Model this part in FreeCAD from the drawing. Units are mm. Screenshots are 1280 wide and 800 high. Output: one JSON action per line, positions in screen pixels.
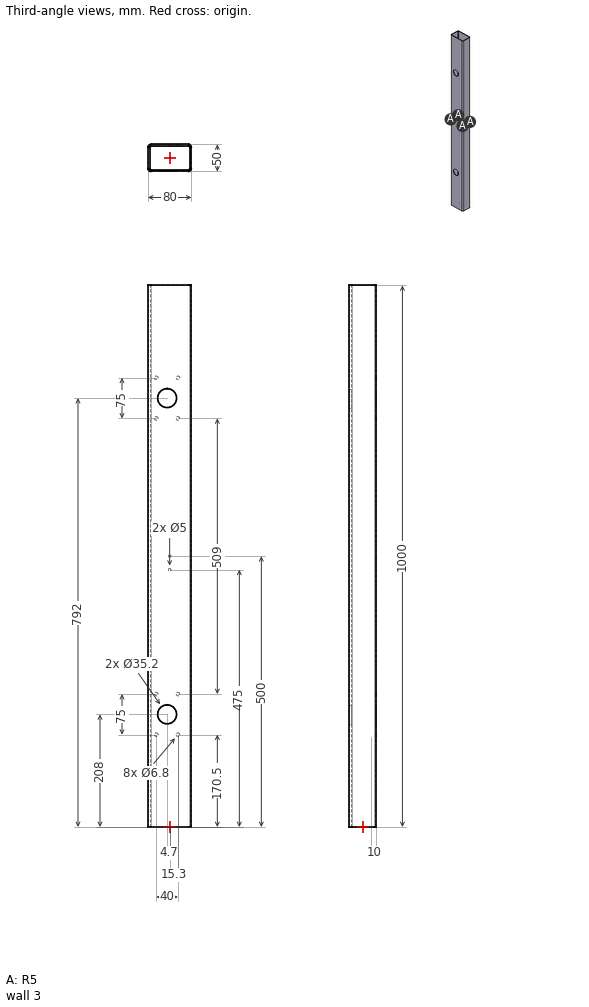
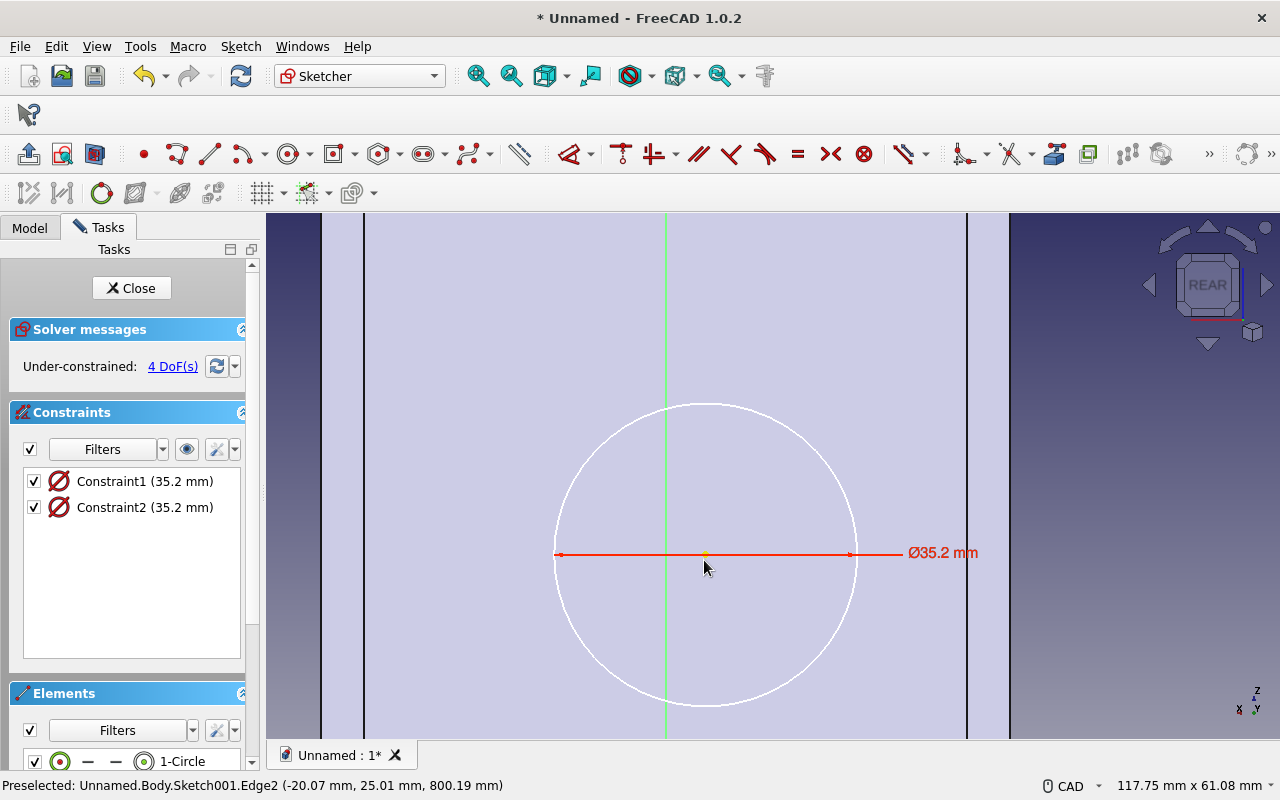
{"action": "left_click", "coordinate": [706, 555]}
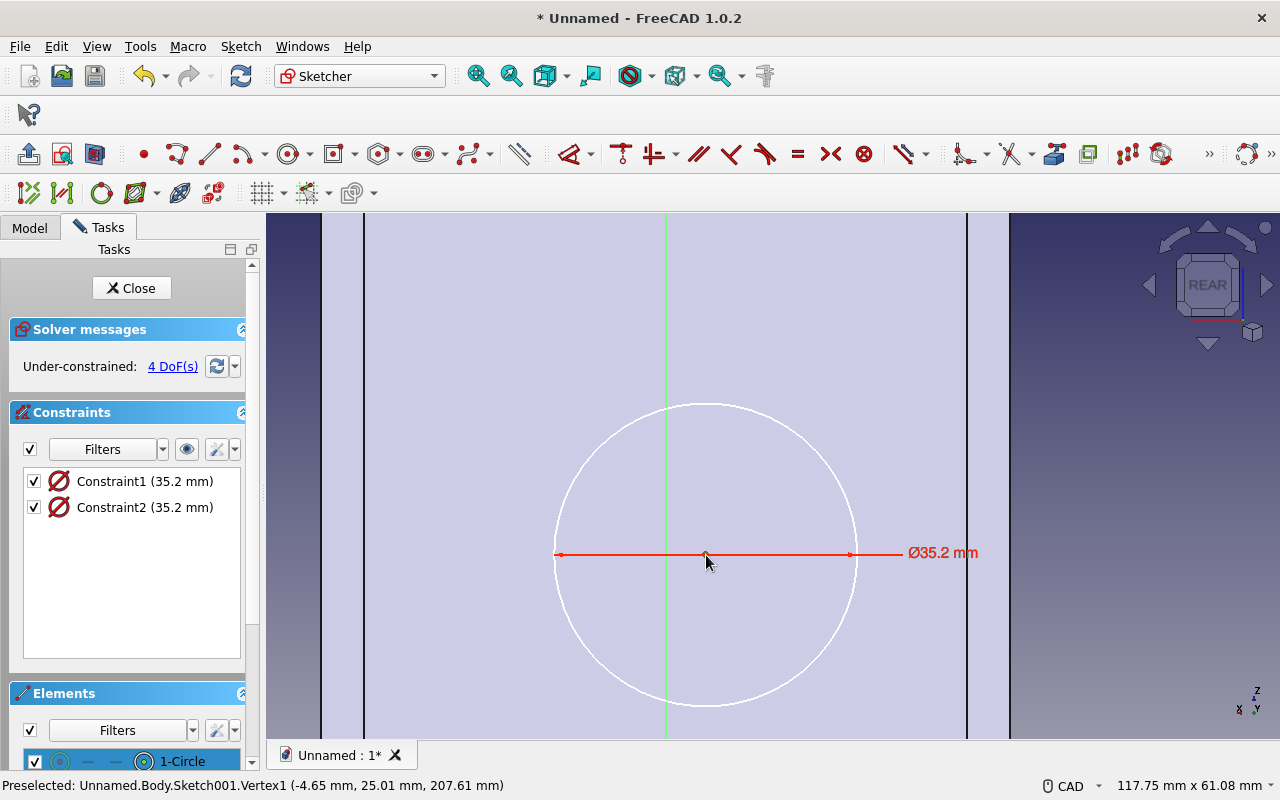
{"action": "key", "text": "l"}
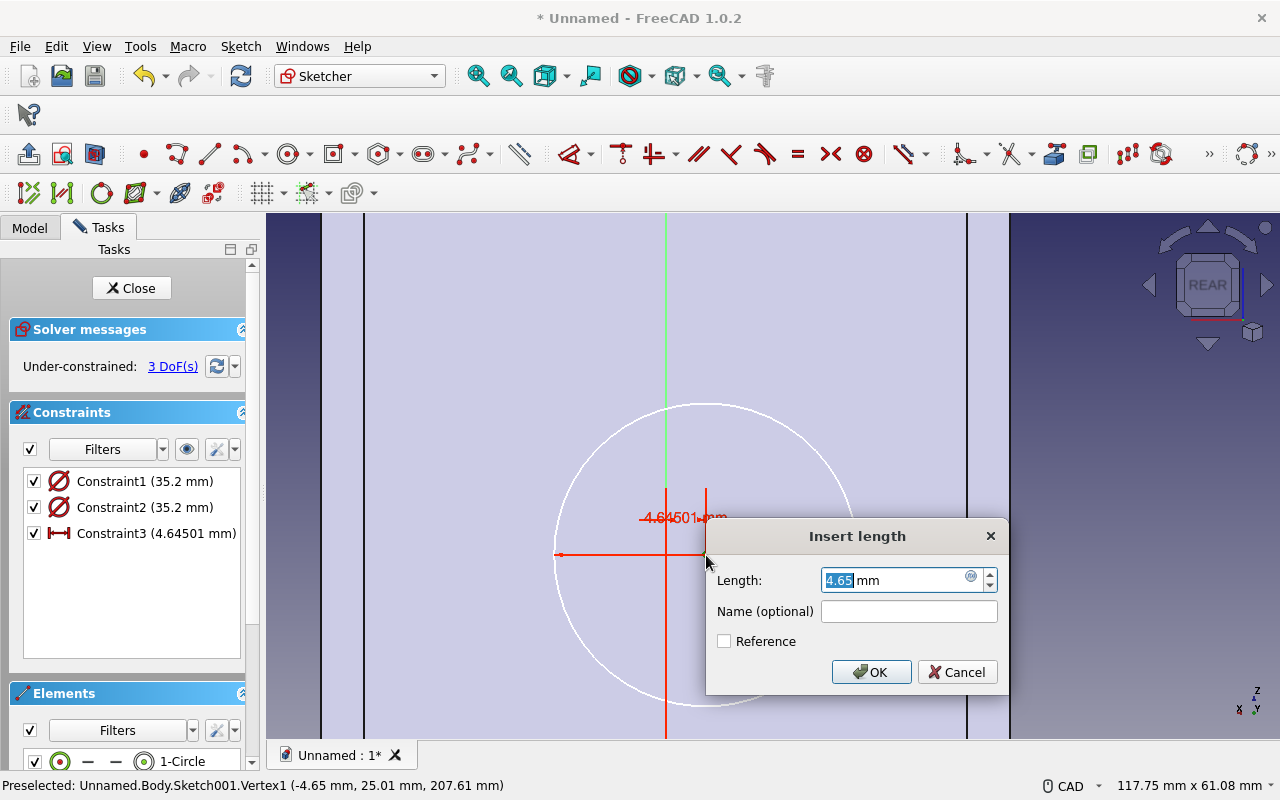
{"action": "type", "text": "4.7"}
{"action": "key", "text": "Return"}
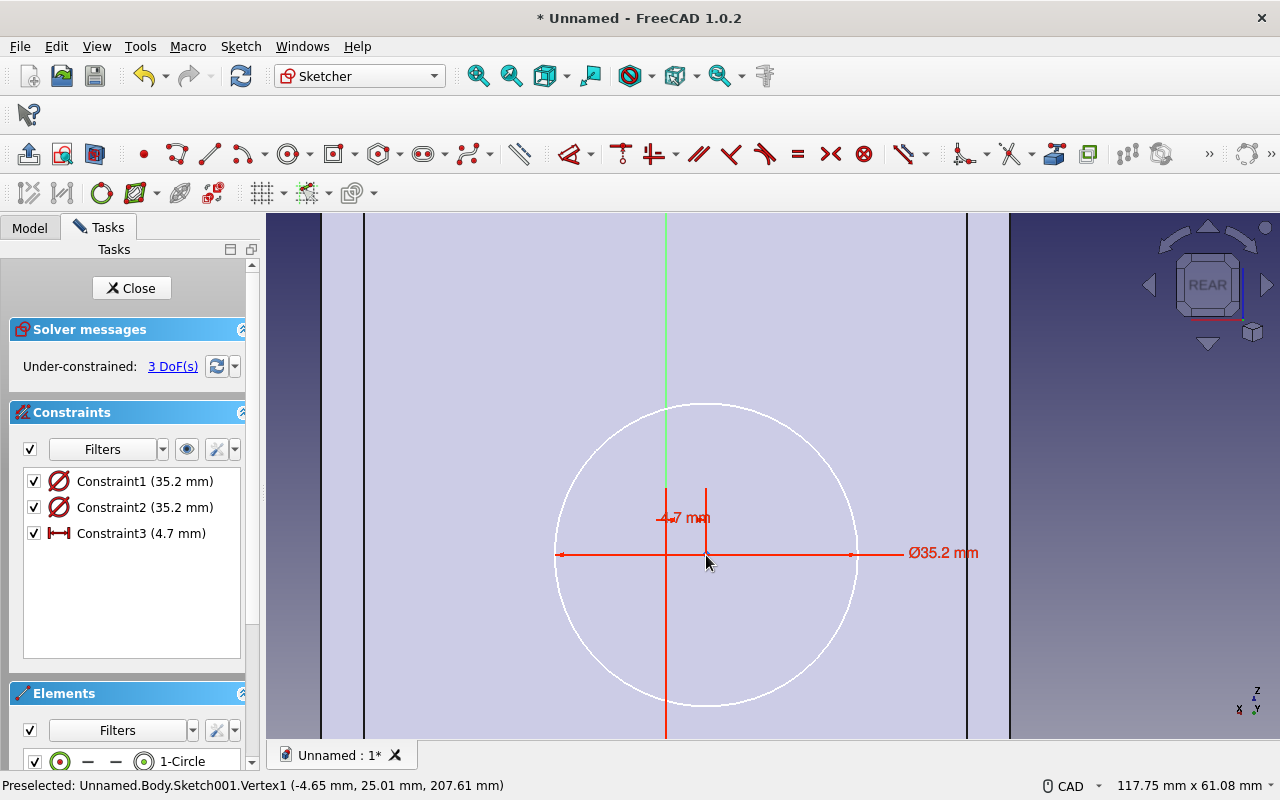
{"action": "scroll", "coordinate": [704, 561], "scroll_direction": "down", "scroll_amount": 15}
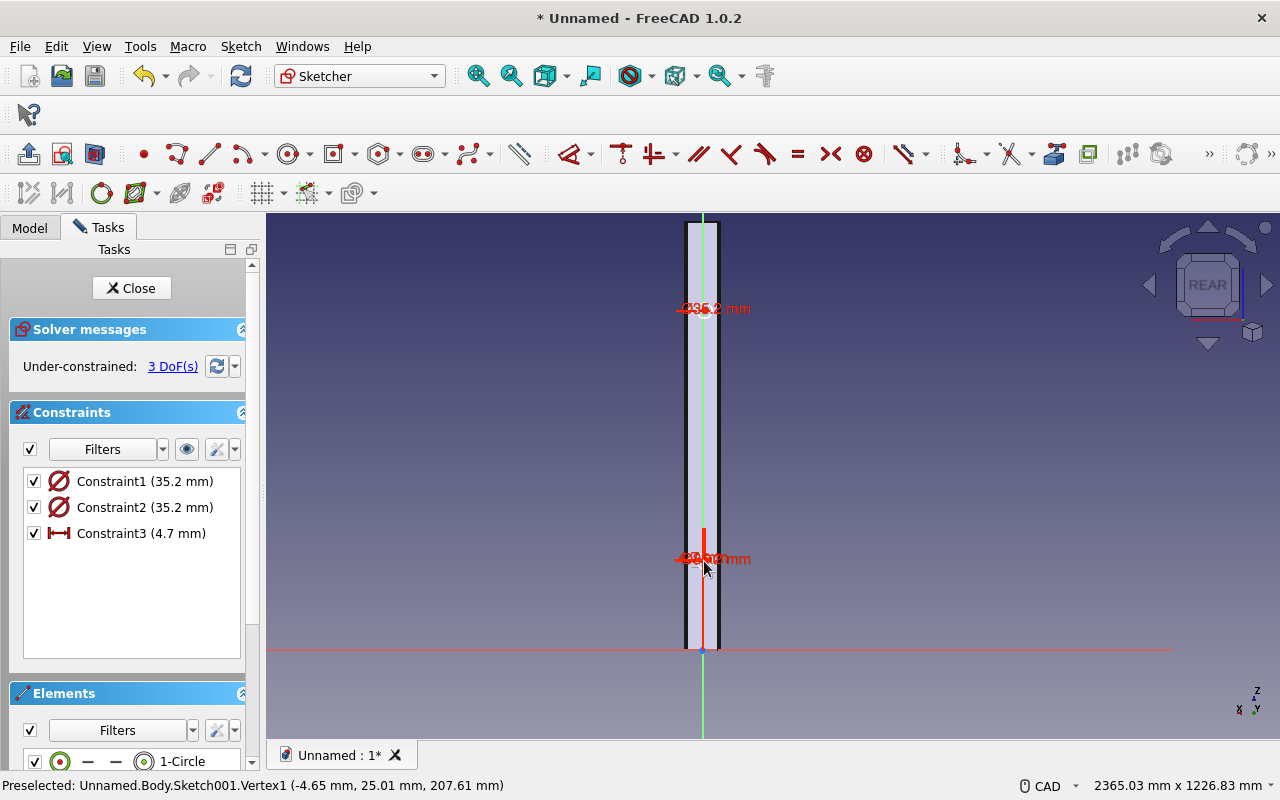
{"action": "left_click", "coordinate": [705, 561]}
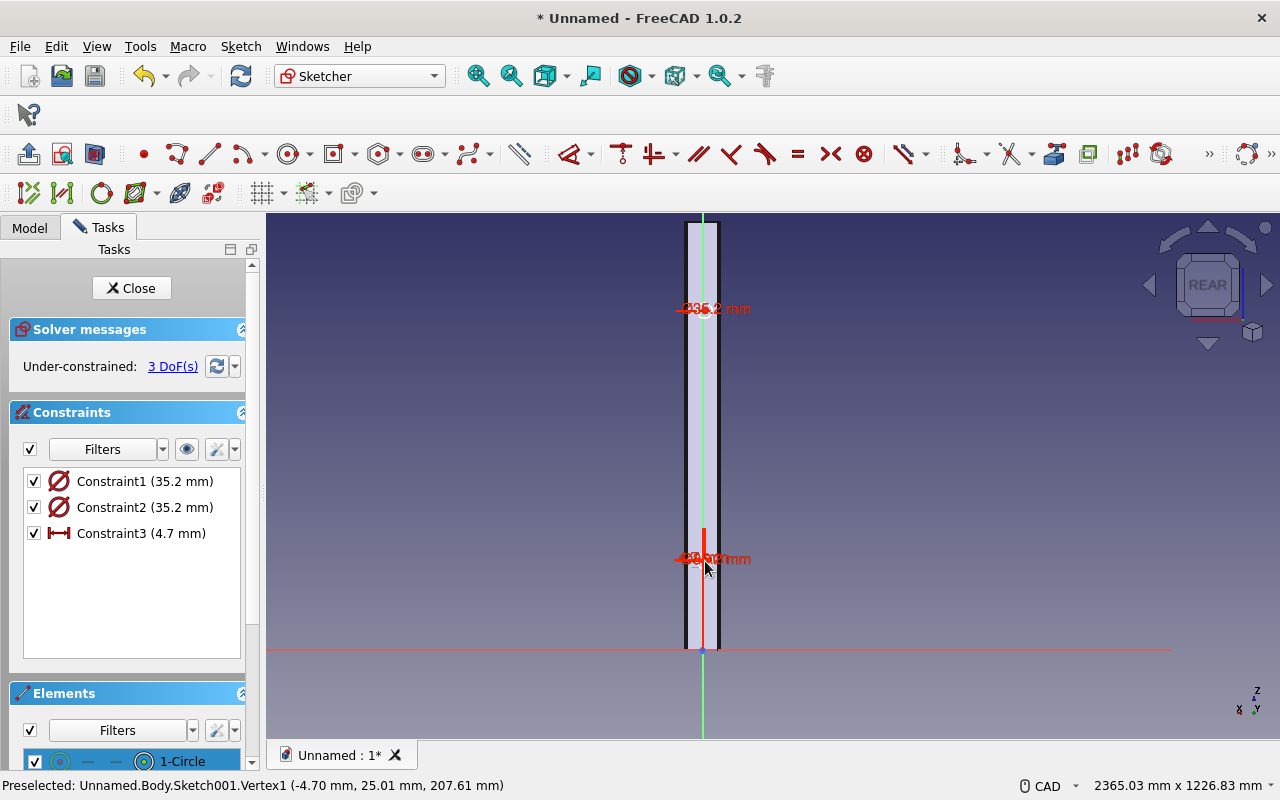
{"action": "left_click", "coordinate": [590, 154]}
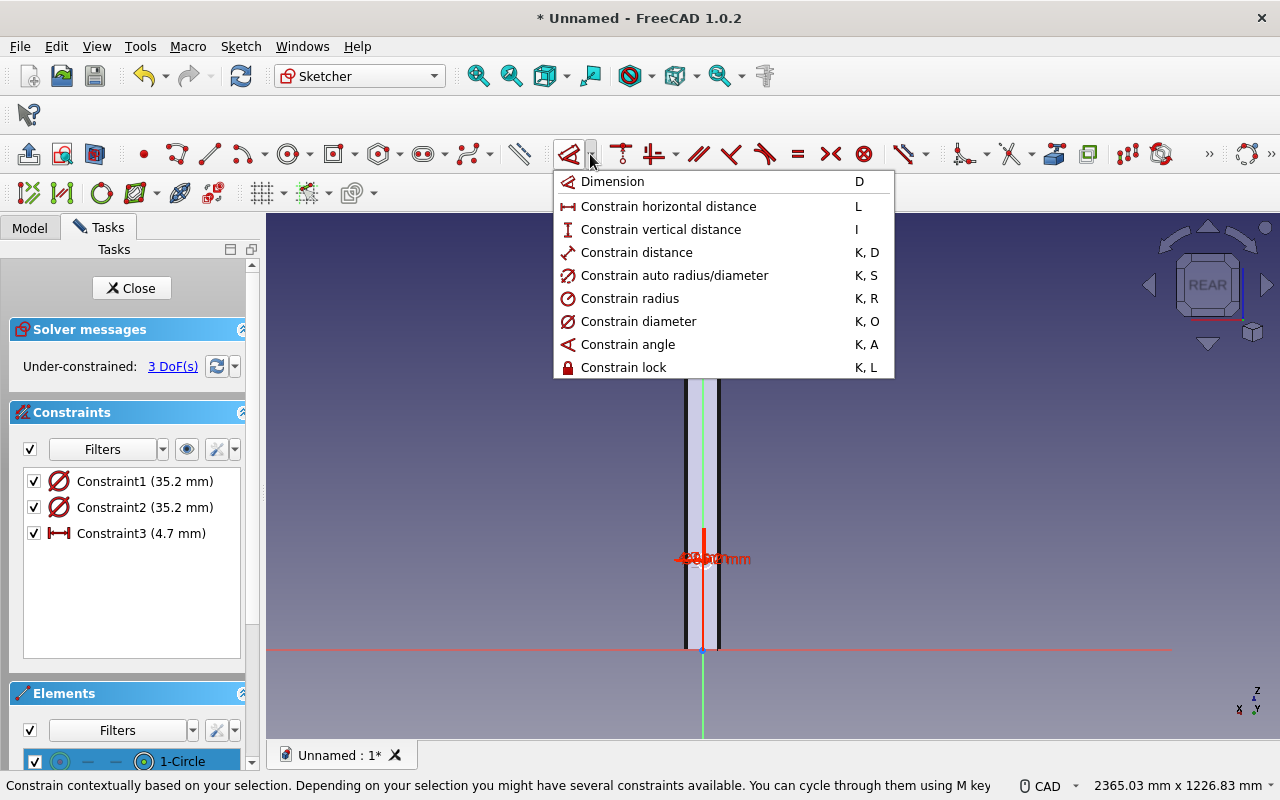
{"action": "left_click", "coordinate": [724, 230]}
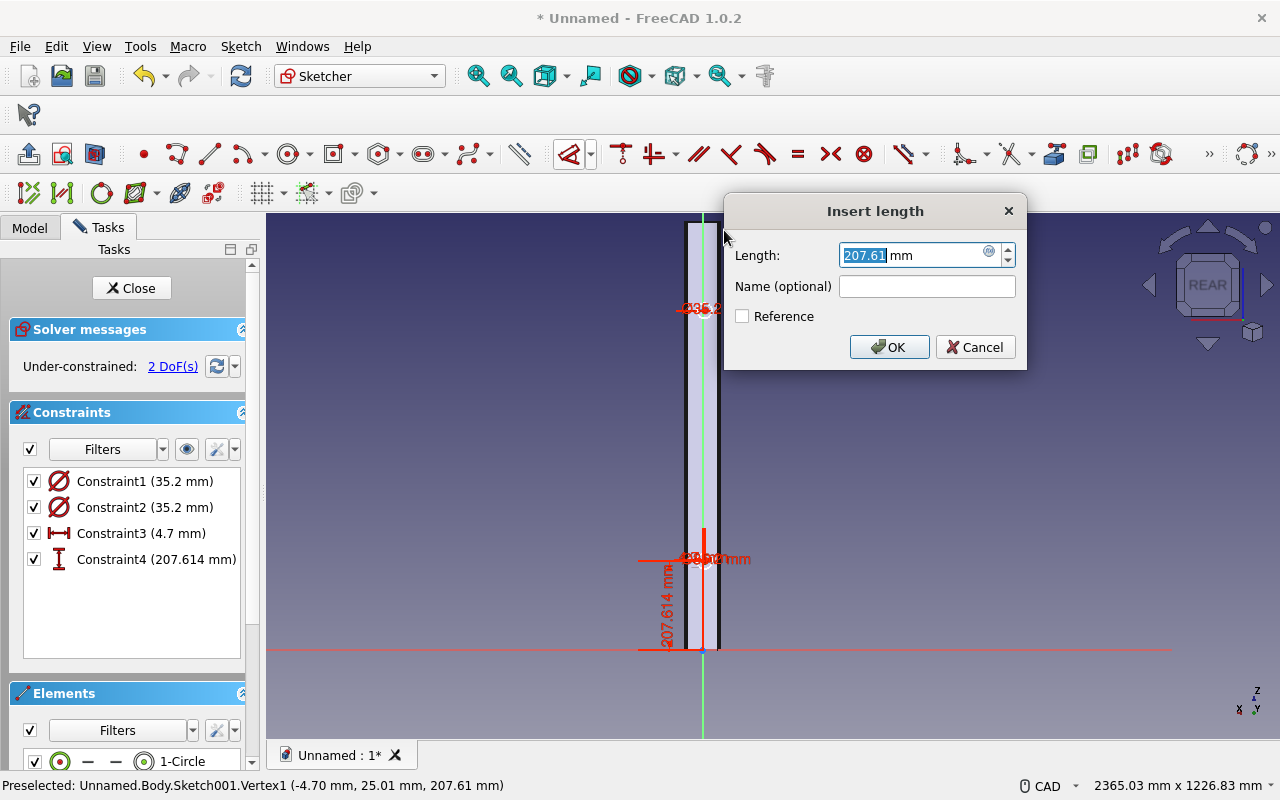
{"action": "type", "text": "208"}
{"action": "key", "text": "Return"}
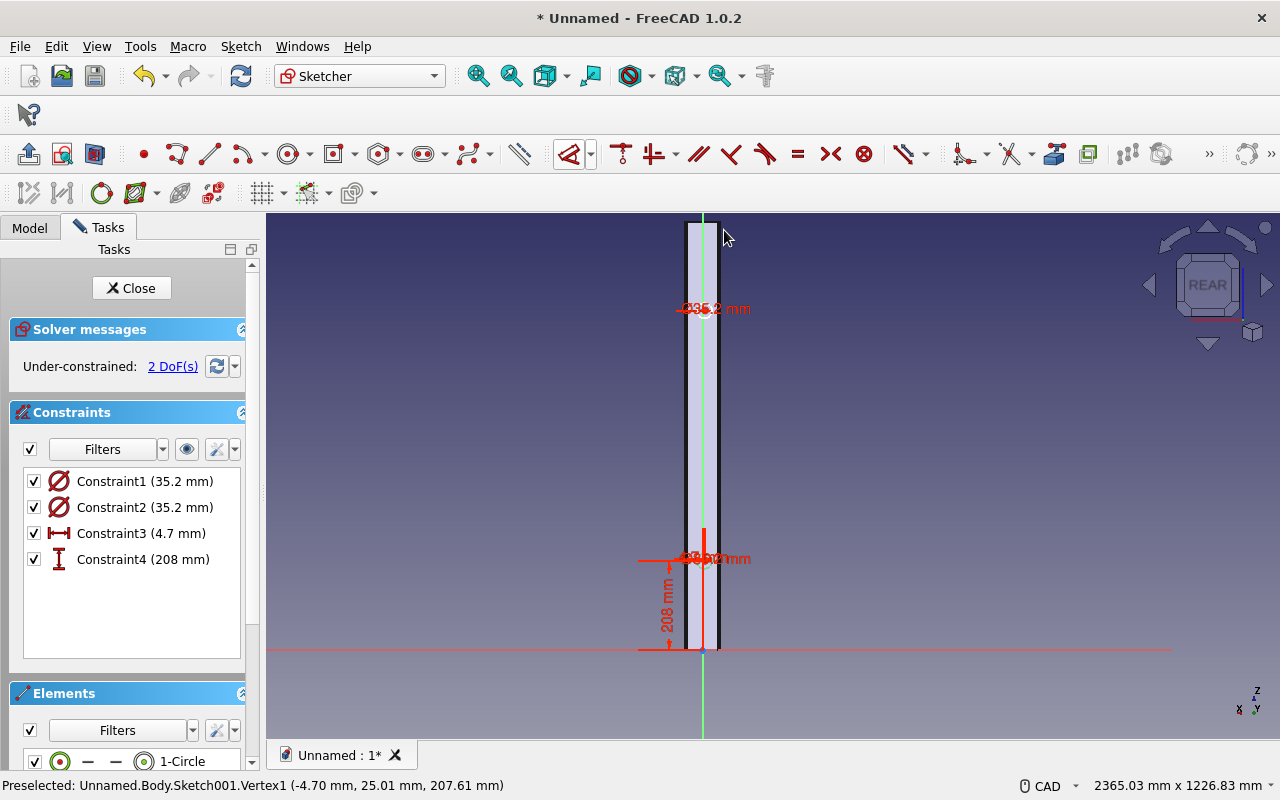
{"action": "scroll", "coordinate": [704, 311], "scroll_direction": "up", "scroll_amount": 15}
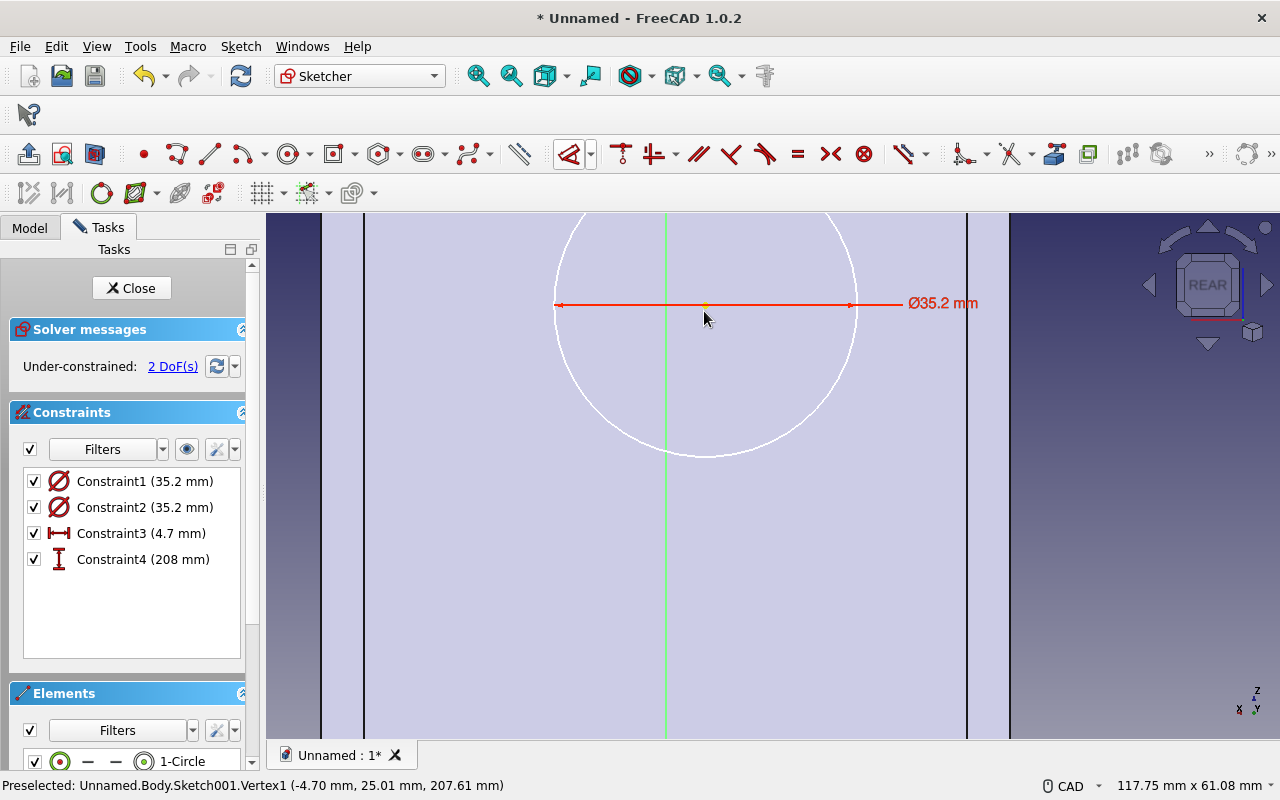
{"action": "left_click", "coordinate": [706, 305]}